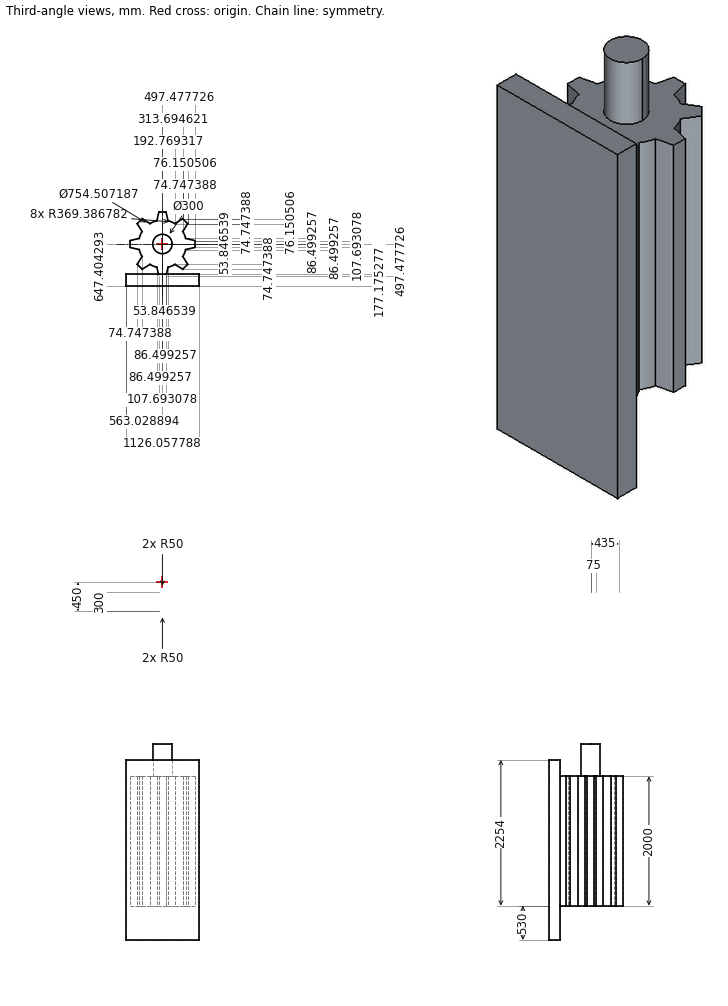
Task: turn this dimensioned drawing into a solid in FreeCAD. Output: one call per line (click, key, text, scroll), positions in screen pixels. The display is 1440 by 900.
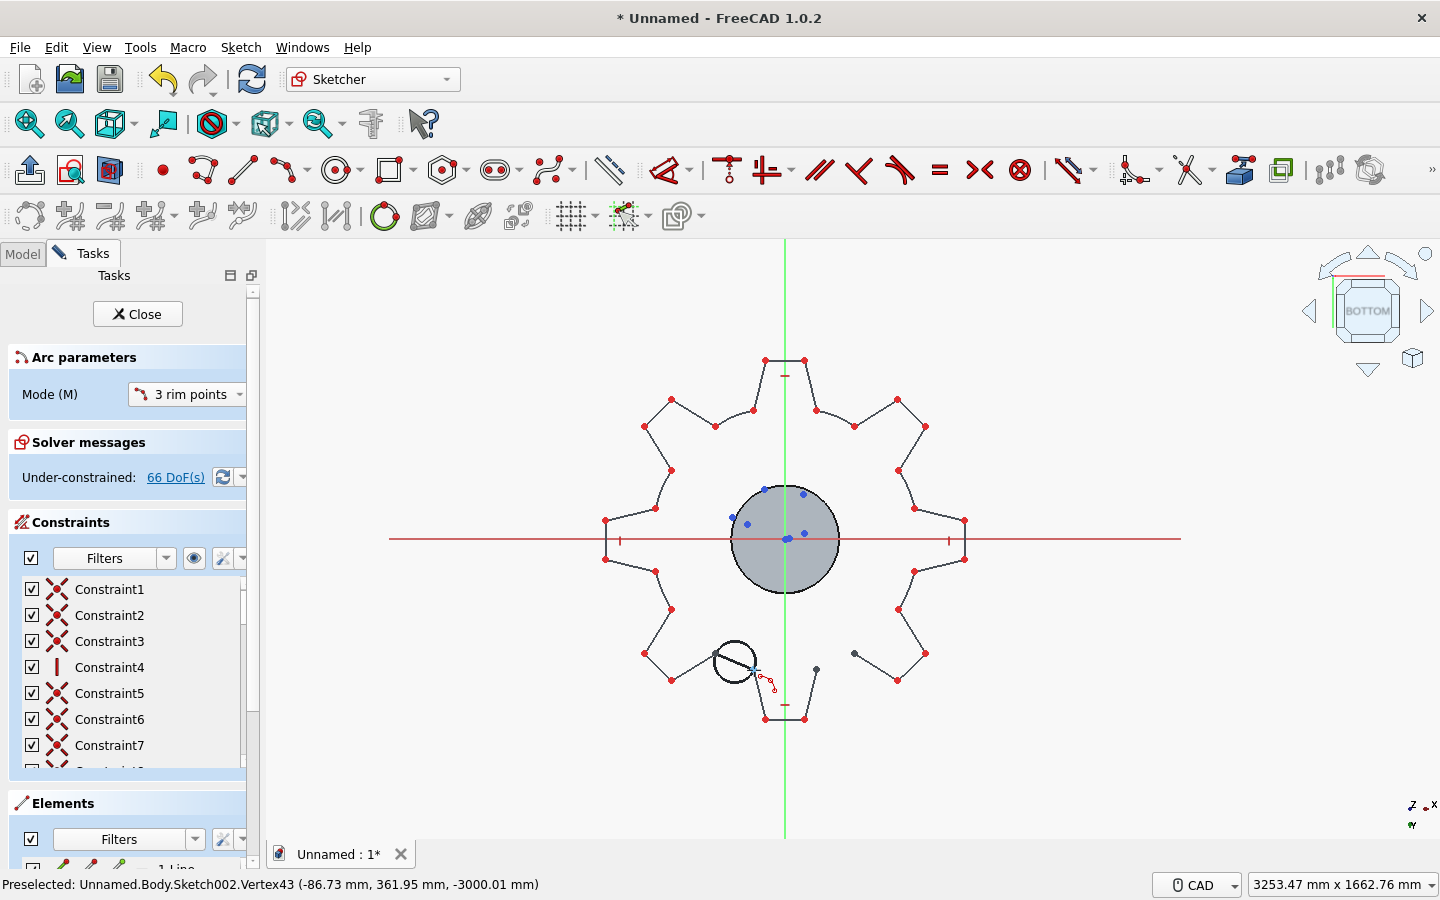
scroll(734, 662, up, 12)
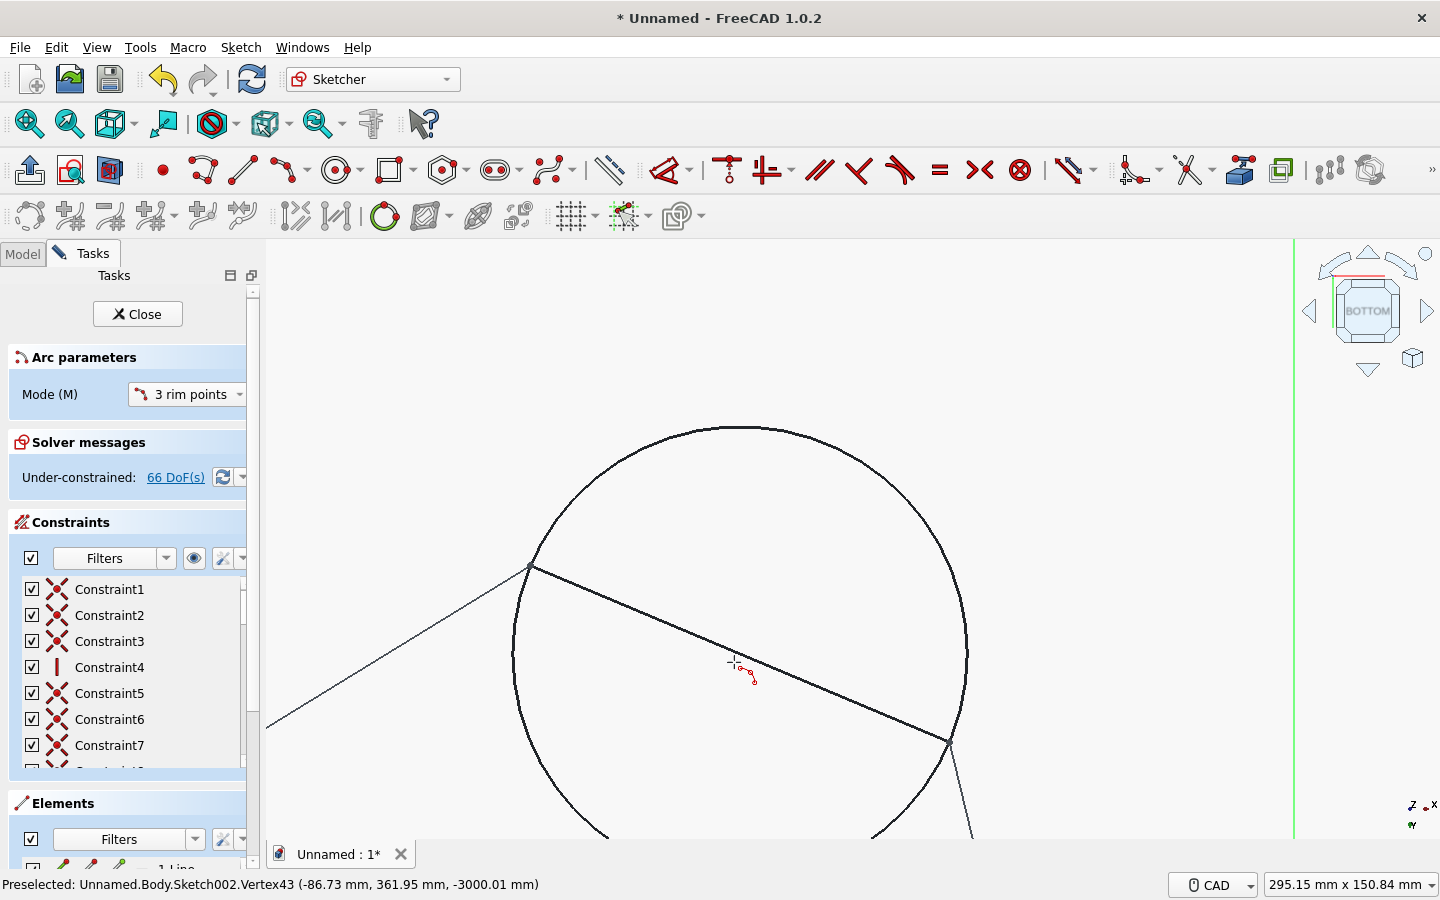
click(732, 660)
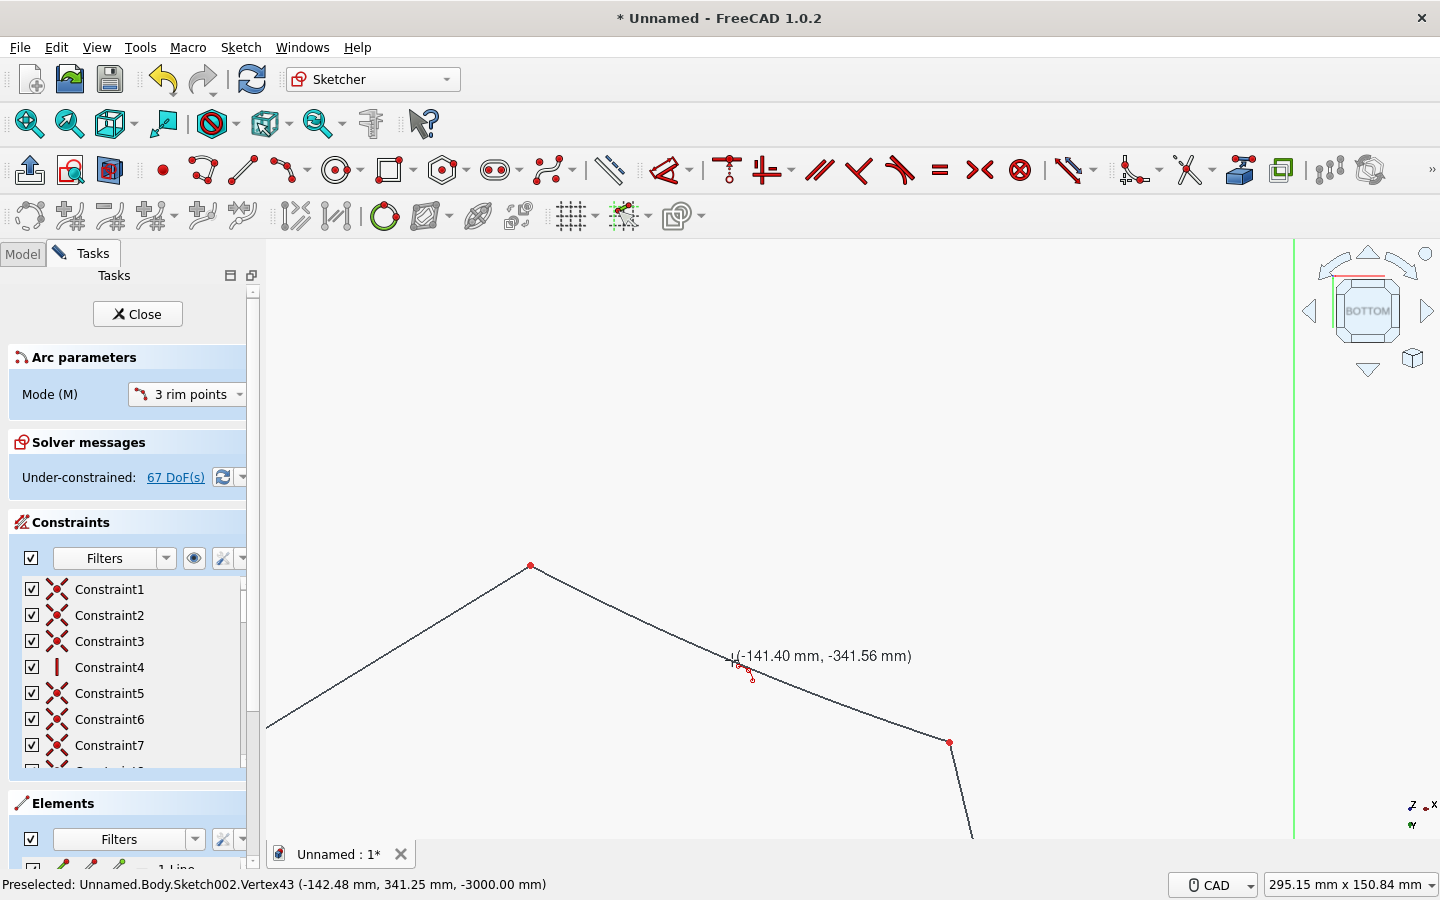
scroll(734, 662, down, 12)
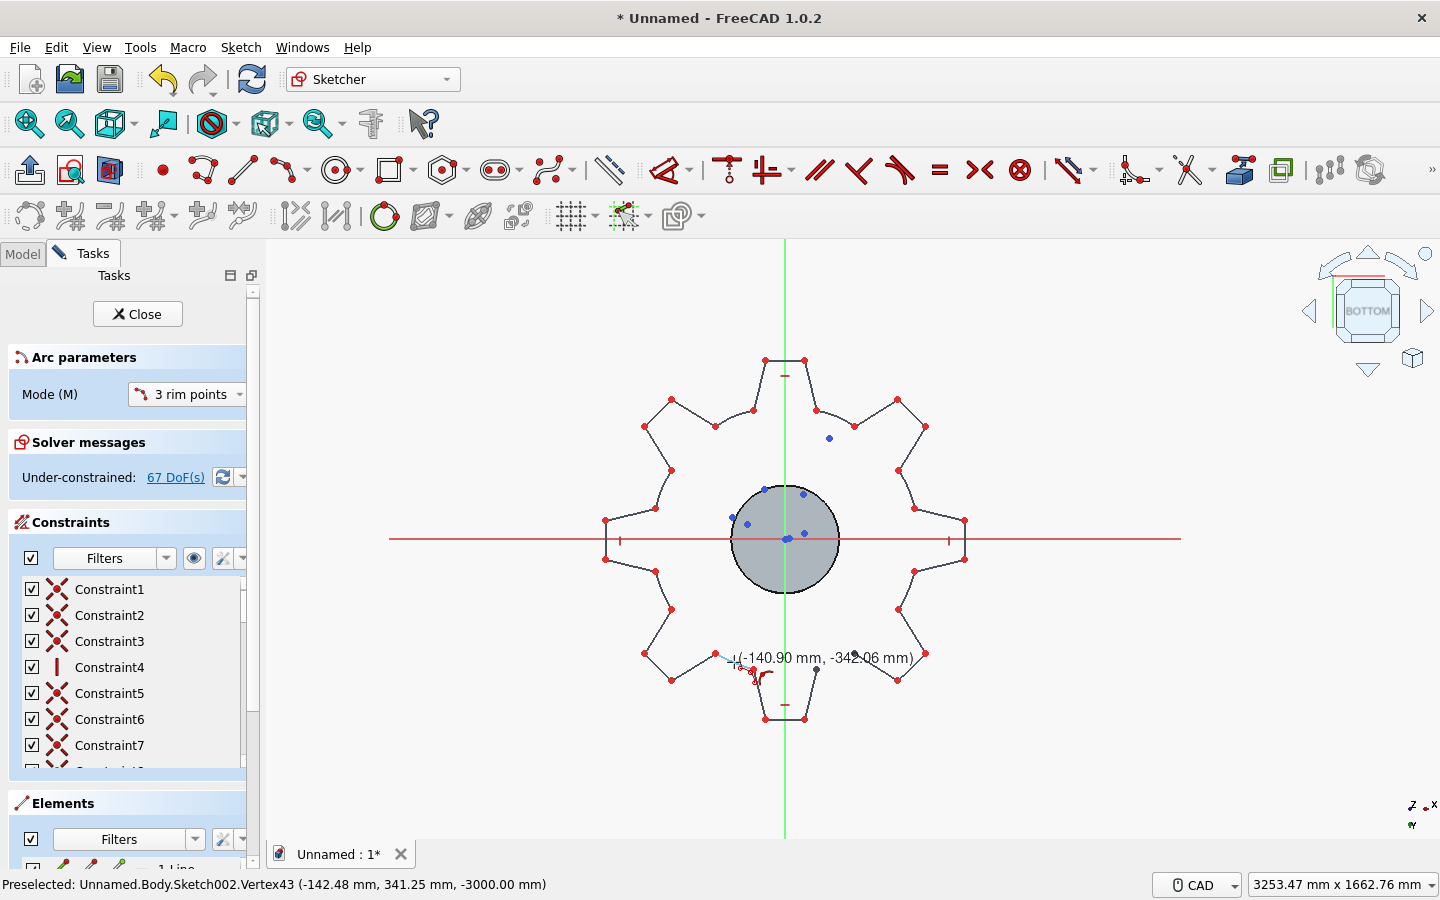
click(817, 670)
click(855, 654)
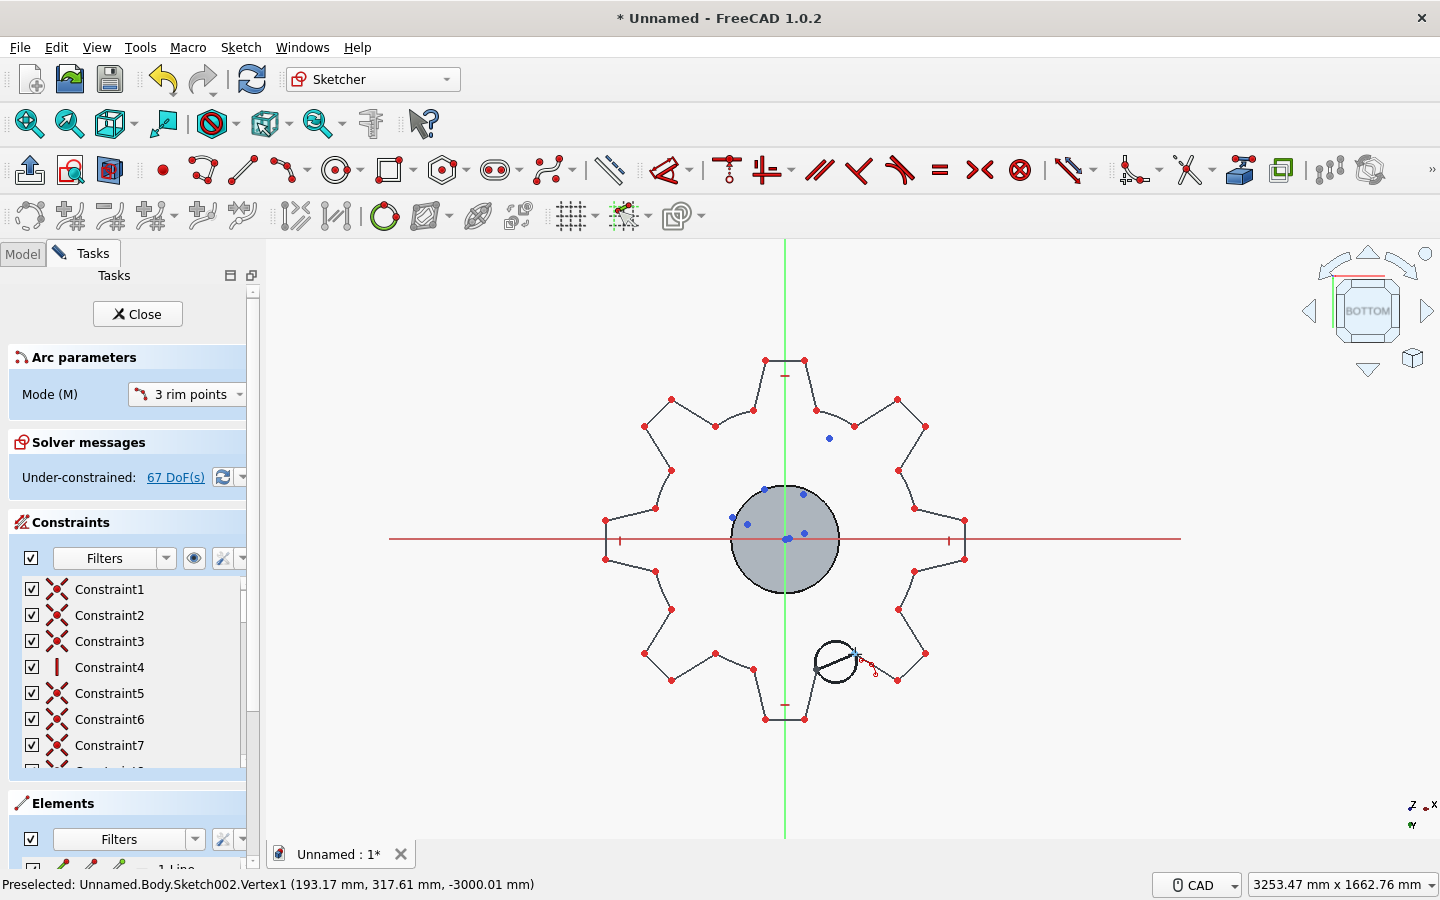
scroll(836, 662, up, 12)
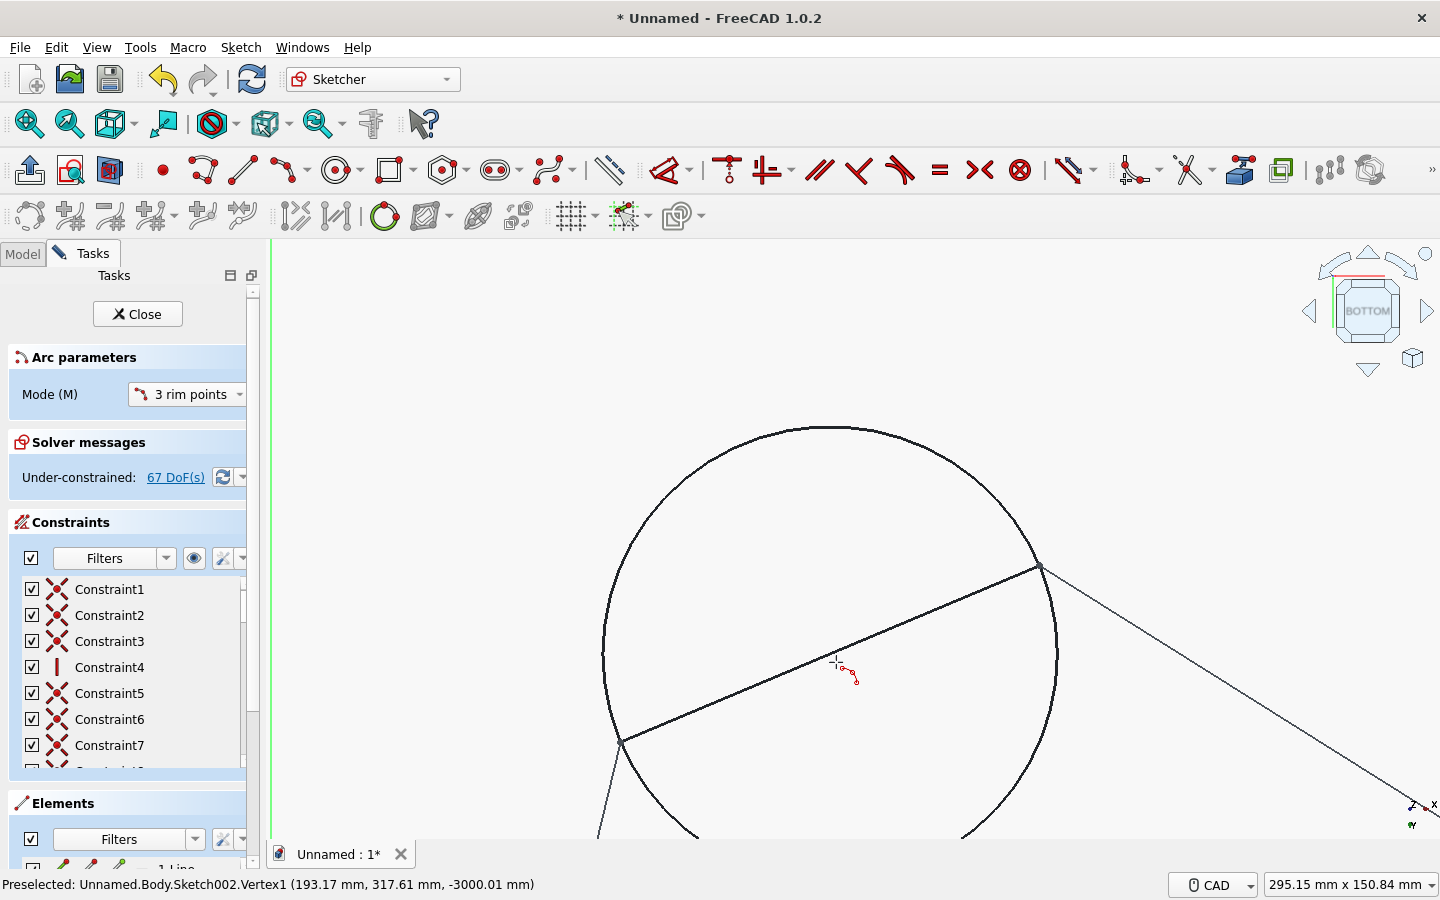
click(833, 660)
key(Escape)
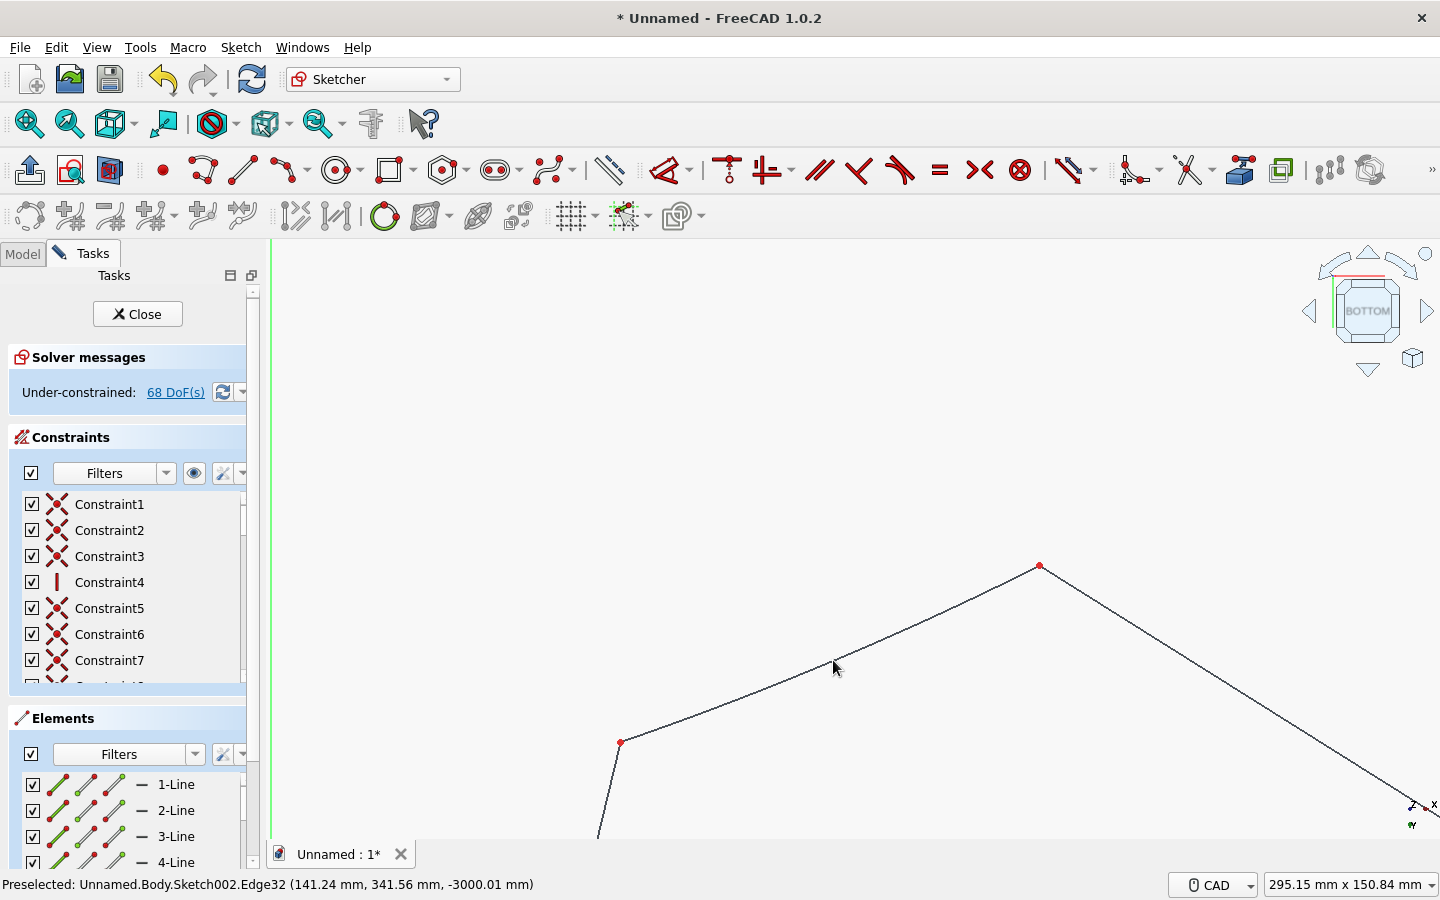
scroll(836, 662, down, 12)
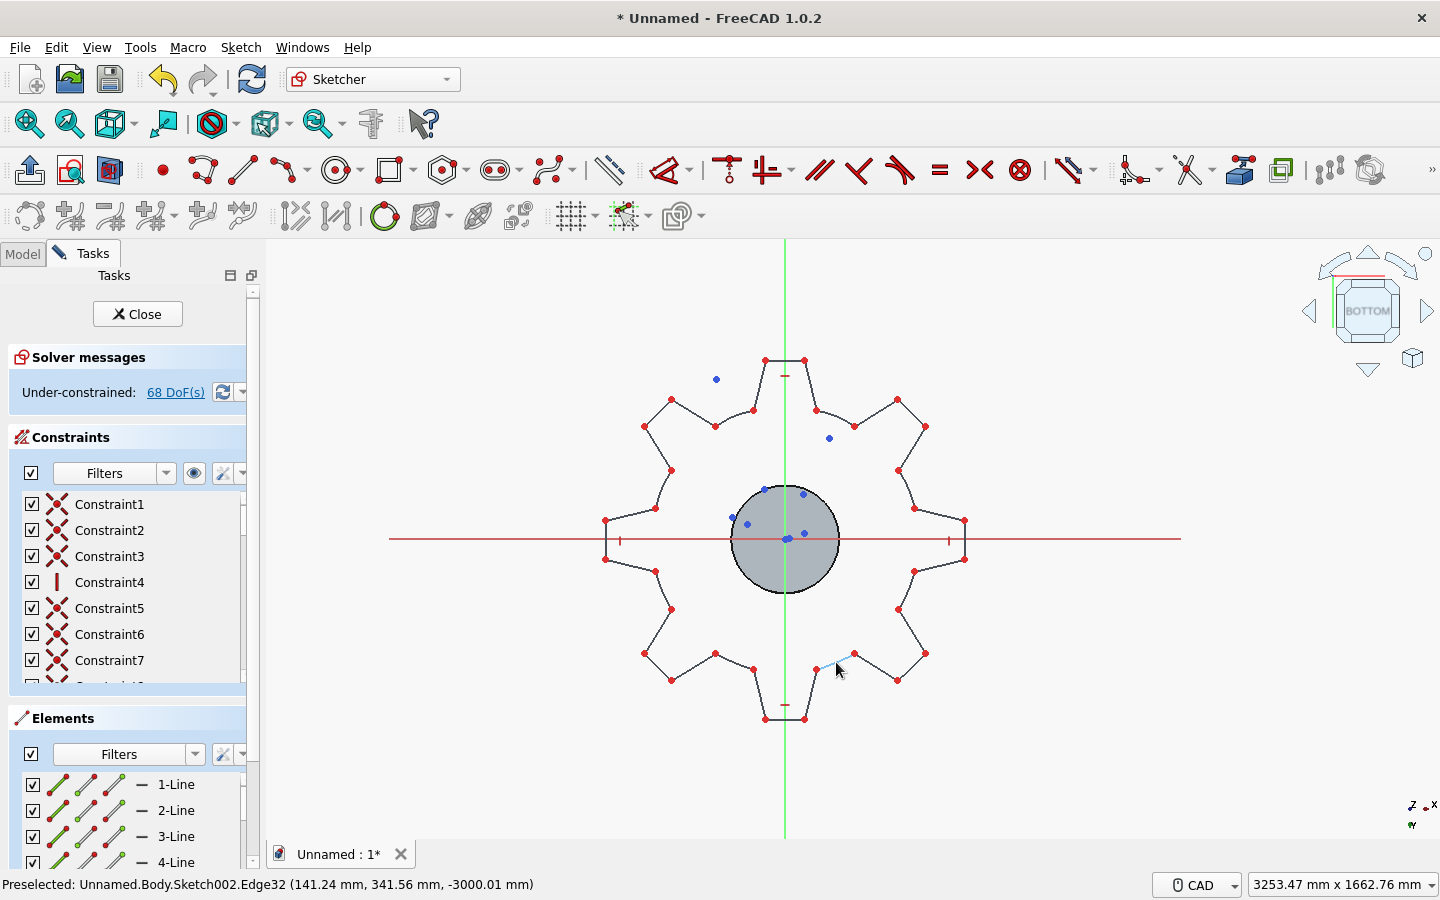
click(905, 599)